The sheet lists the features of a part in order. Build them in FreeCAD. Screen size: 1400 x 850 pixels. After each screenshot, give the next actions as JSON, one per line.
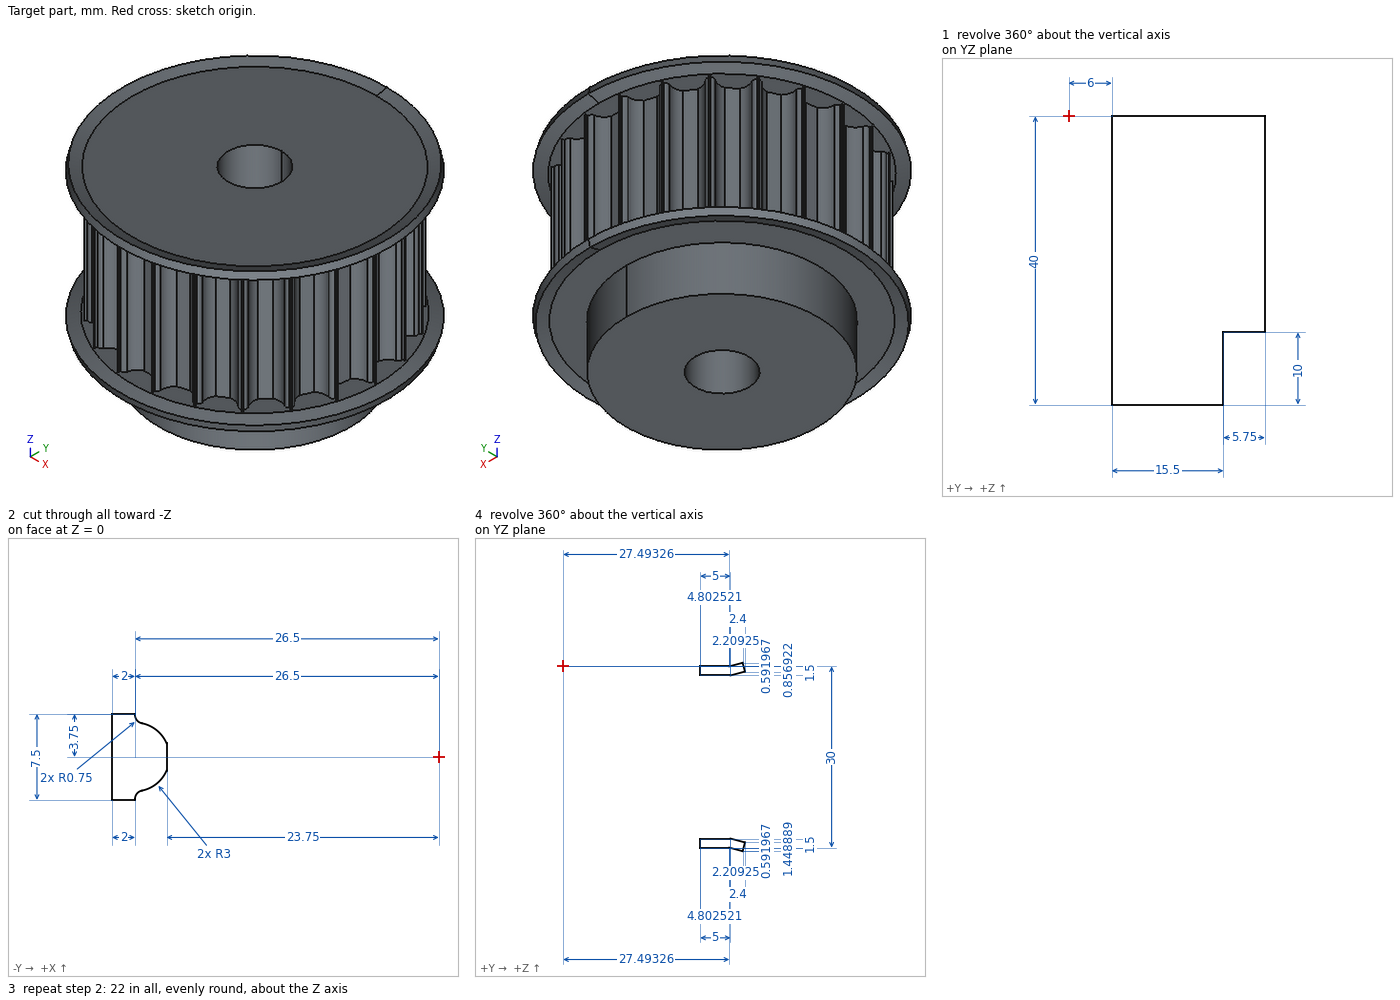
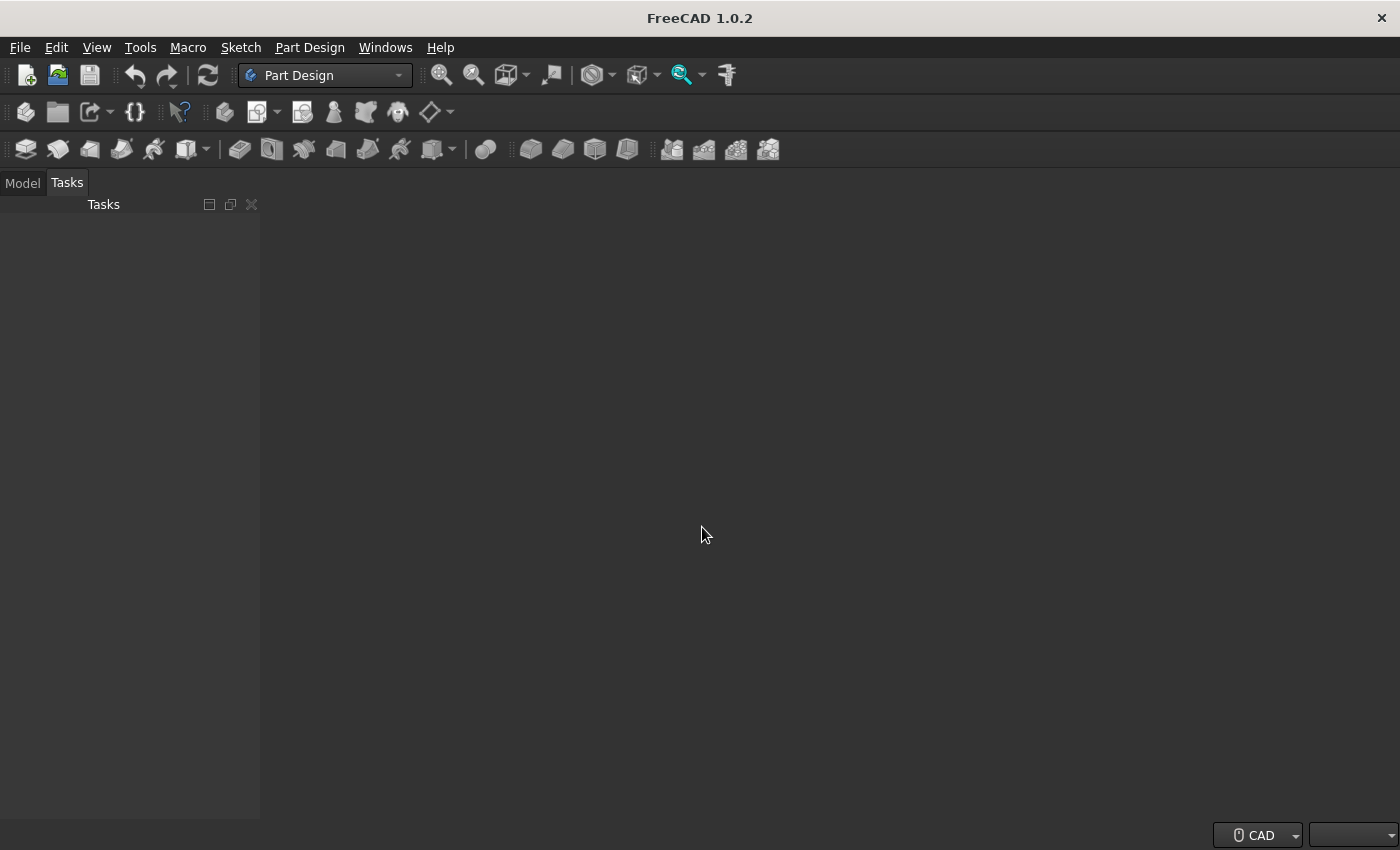
{"action": "left_click", "coordinate": [26, 76]}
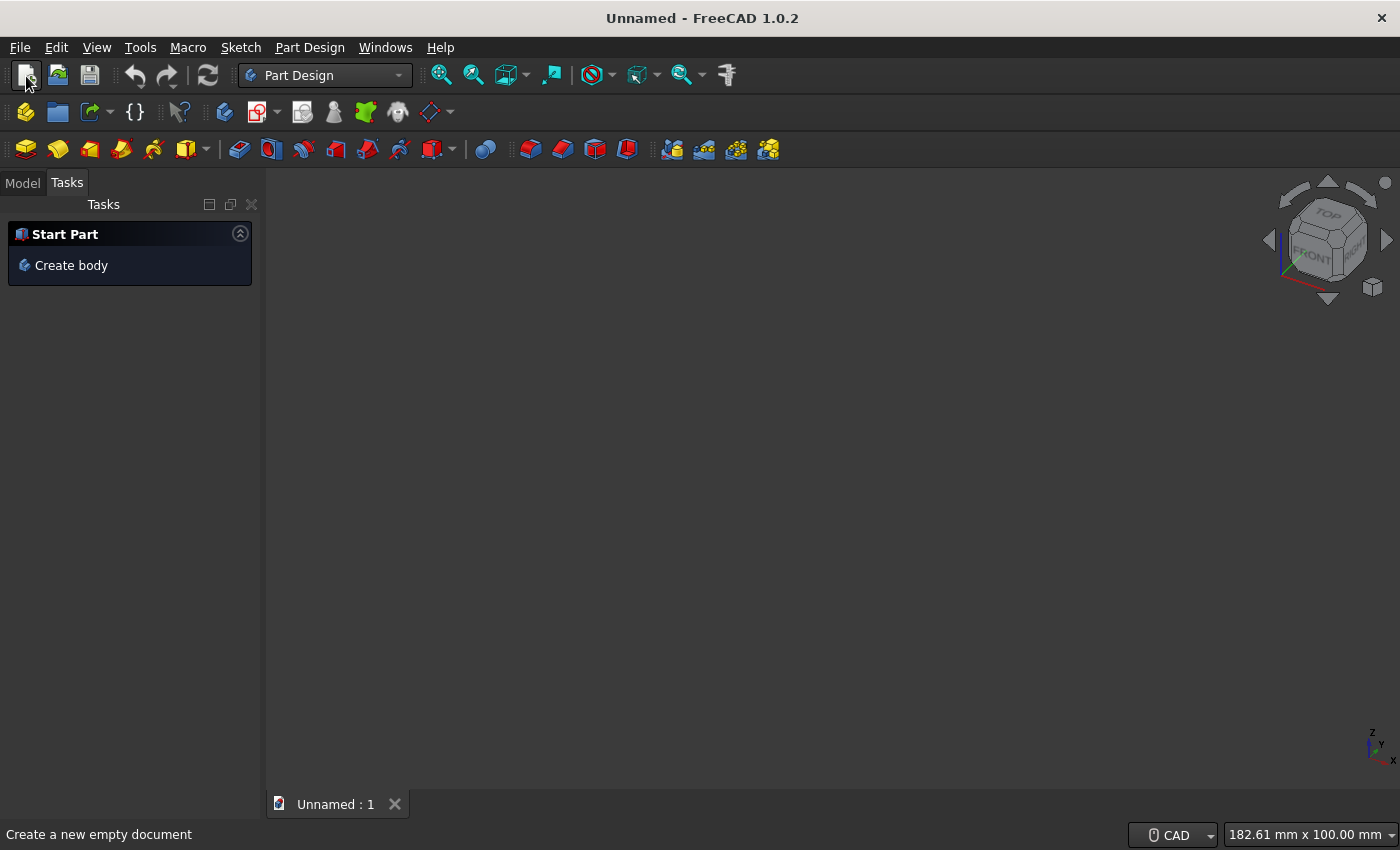
{"action": "left_click", "coordinate": [258, 112]}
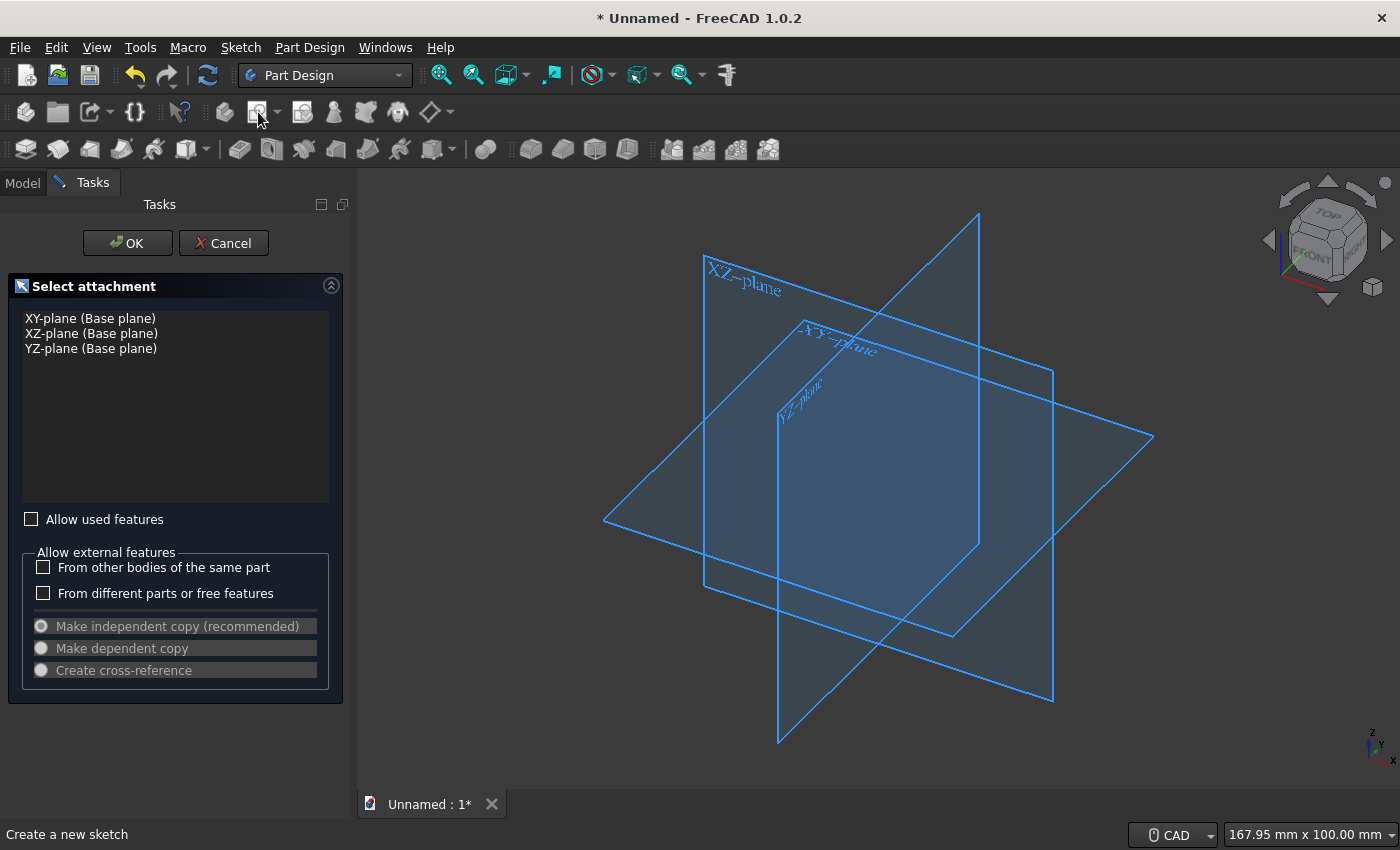
{"action": "left_click", "coordinate": [82, 348]}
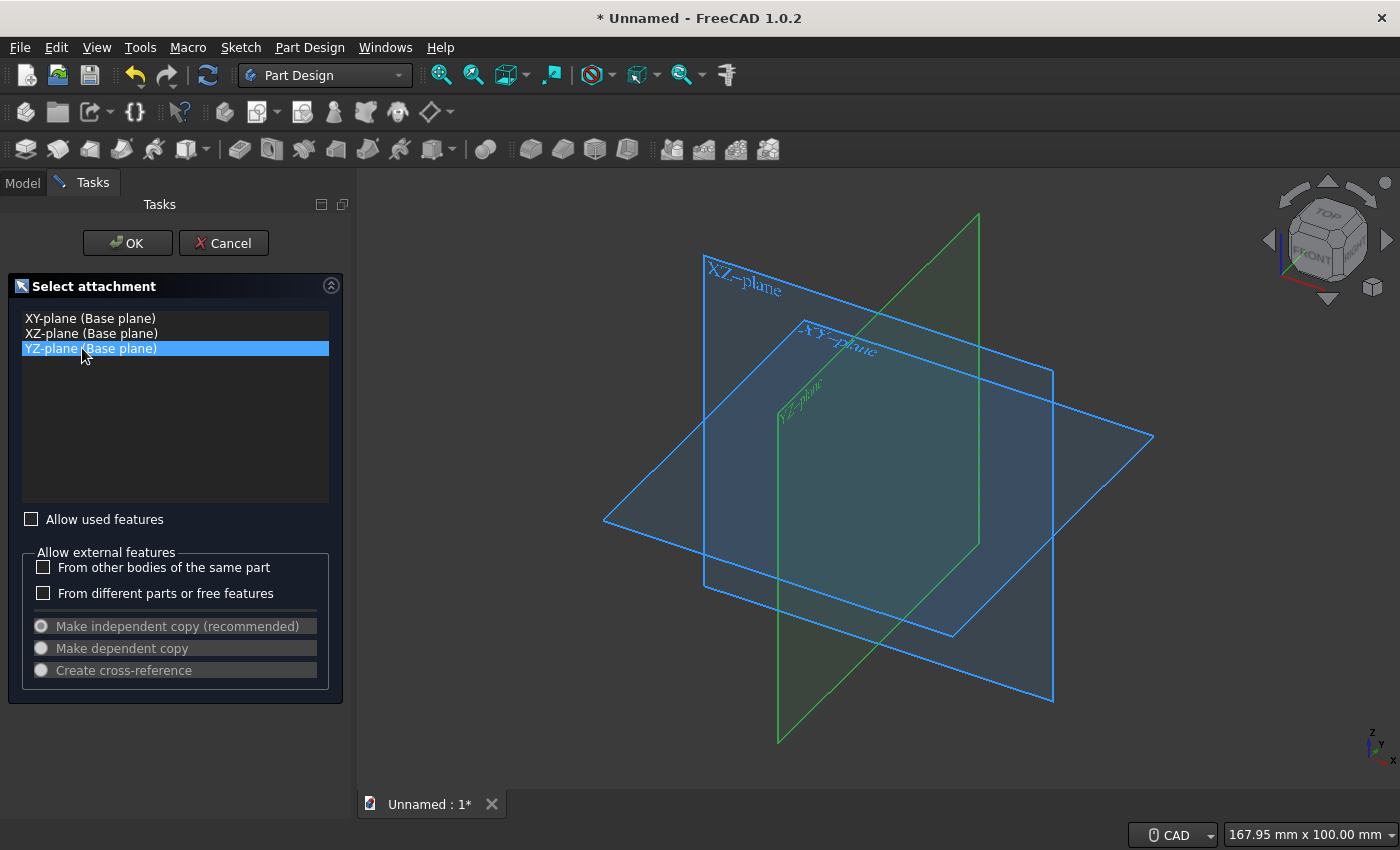
{"action": "left_click", "coordinate": [128, 243]}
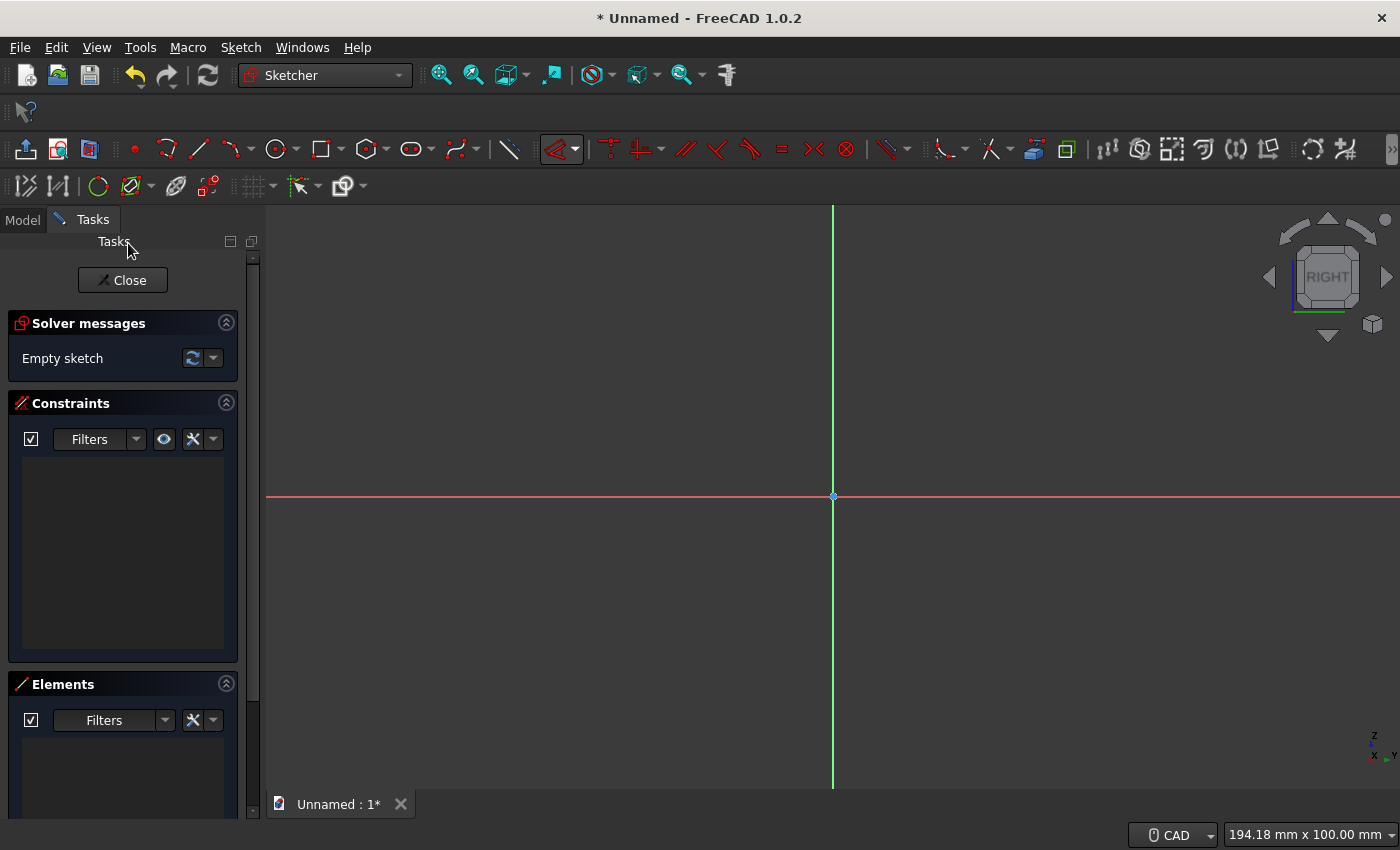
{"action": "scroll", "coordinate": [1214, 761], "scroll_direction": "up", "scroll_amount": 2}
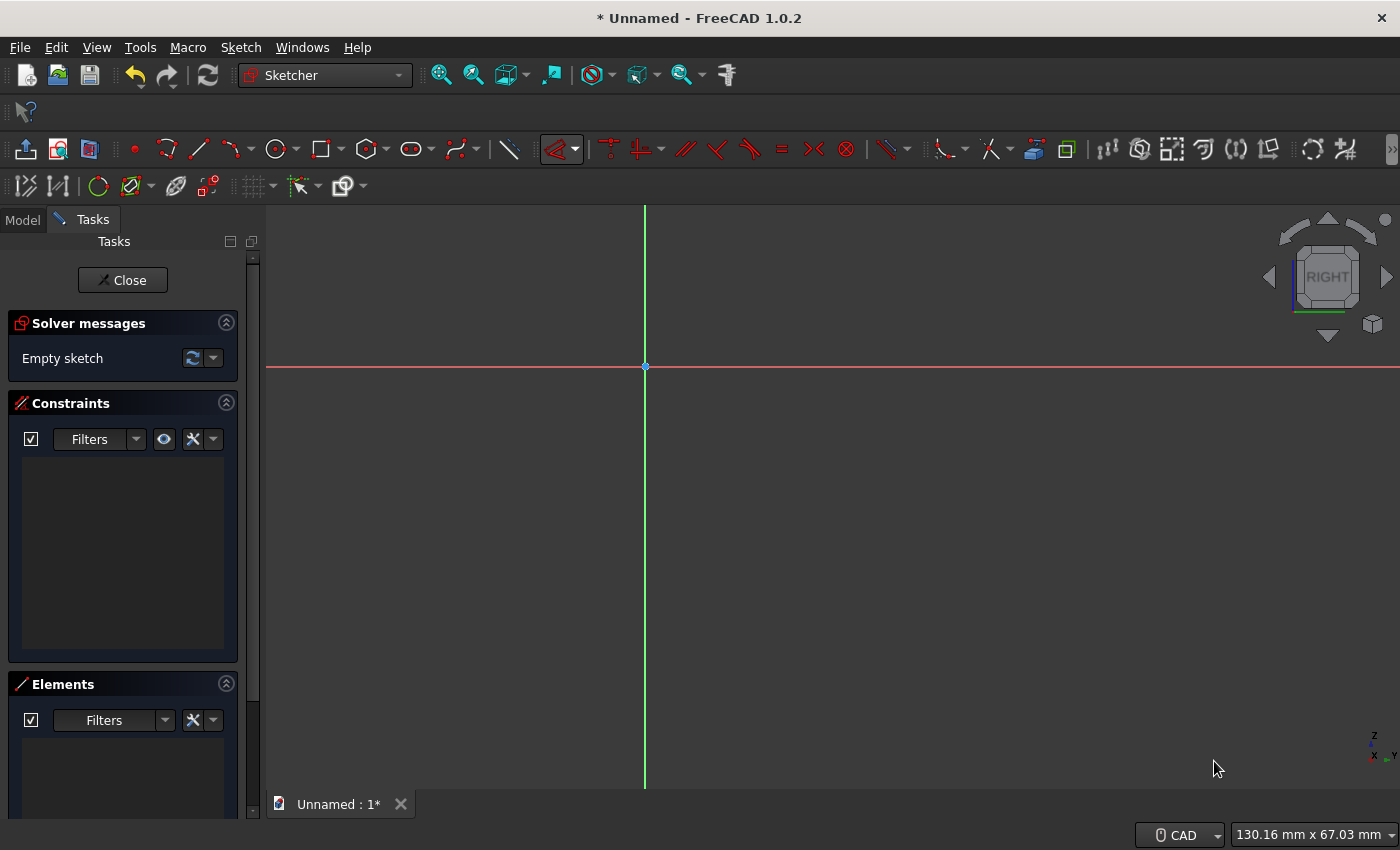
{"action": "left_click", "coordinate": [168, 150]}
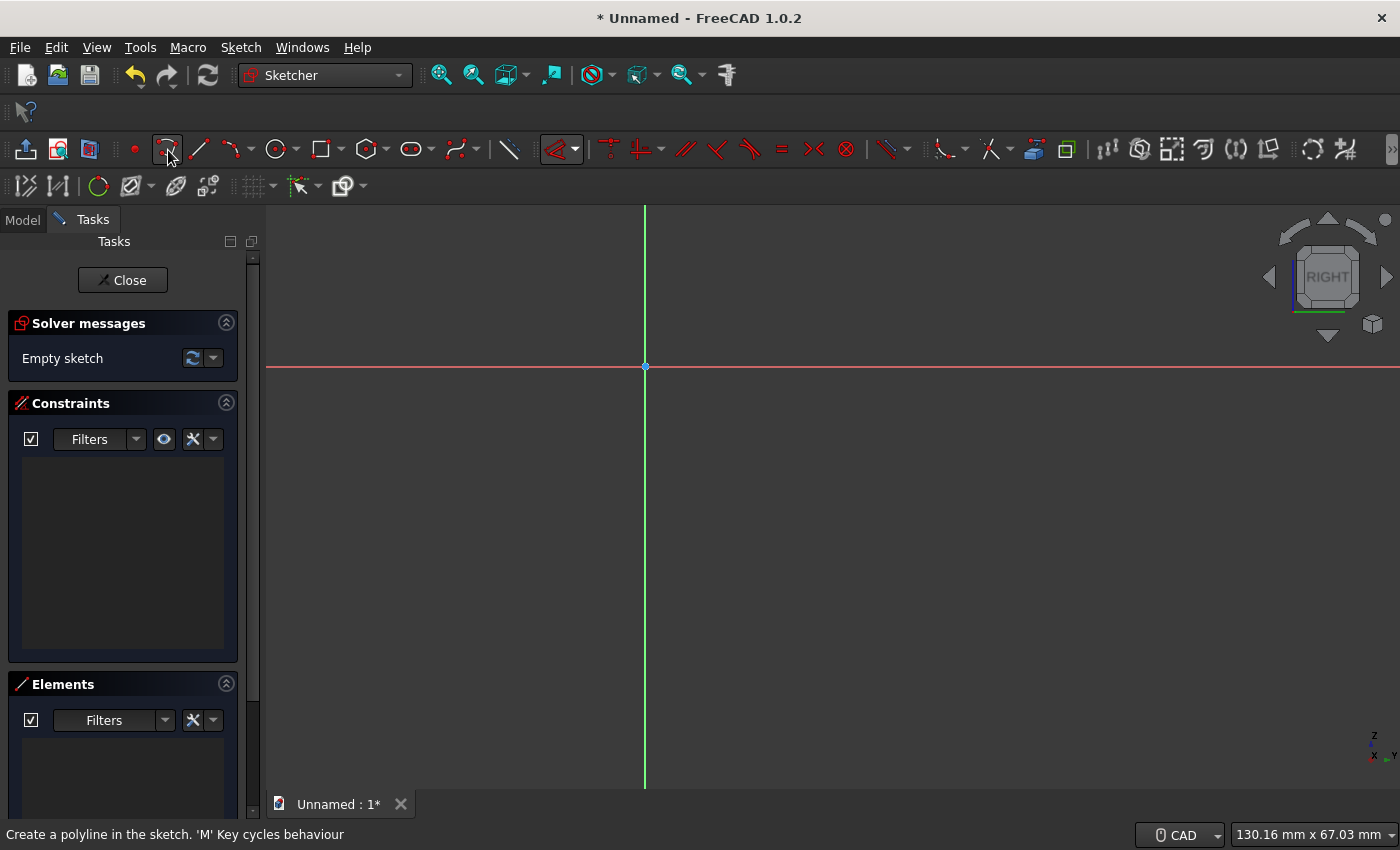
{"action": "left_click", "coordinate": [697, 367]}
{"action": "left_click", "coordinate": [697, 715]}
{"action": "left_click", "coordinate": [833, 715]}
{"action": "left_click", "coordinate": [833, 628]}
{"action": "left_click", "coordinate": [883, 628]}
{"action": "left_click", "coordinate": [883, 376]}
{"action": "left_click", "coordinate": [697, 367]}
{"action": "key", "text": "Escape"}
{"action": "key", "text": "Escape"}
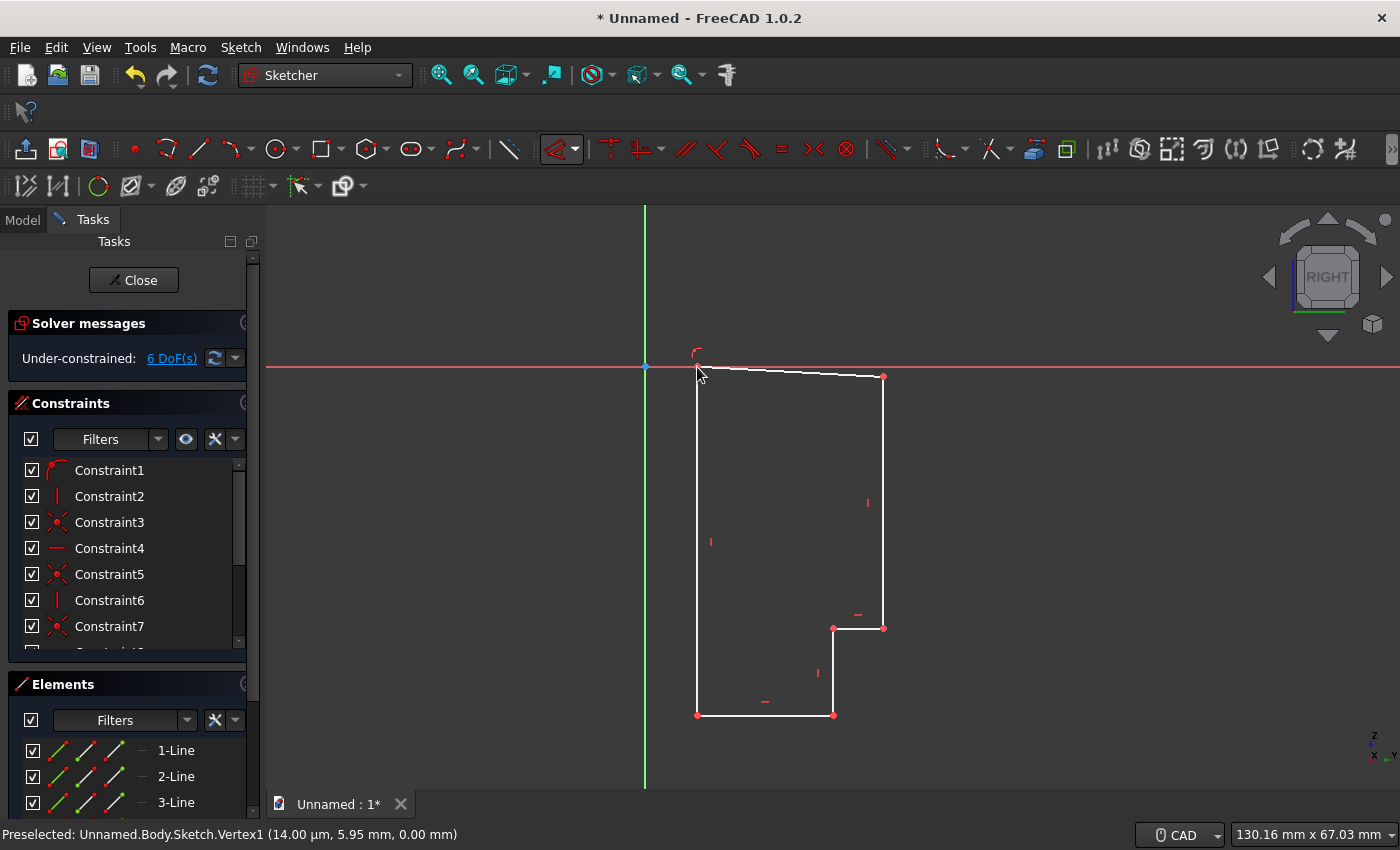
{"action": "left_click", "coordinate": [753, 370]}